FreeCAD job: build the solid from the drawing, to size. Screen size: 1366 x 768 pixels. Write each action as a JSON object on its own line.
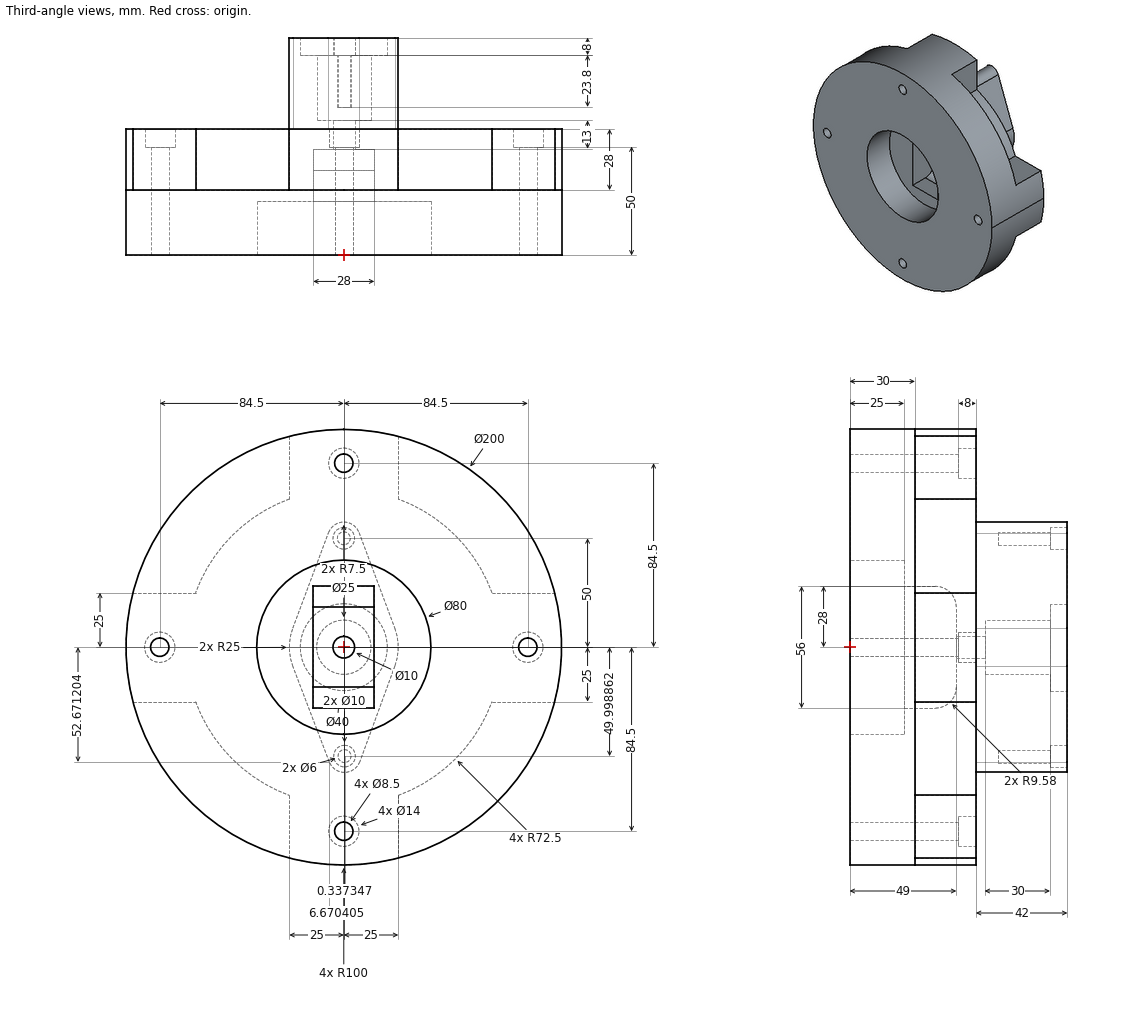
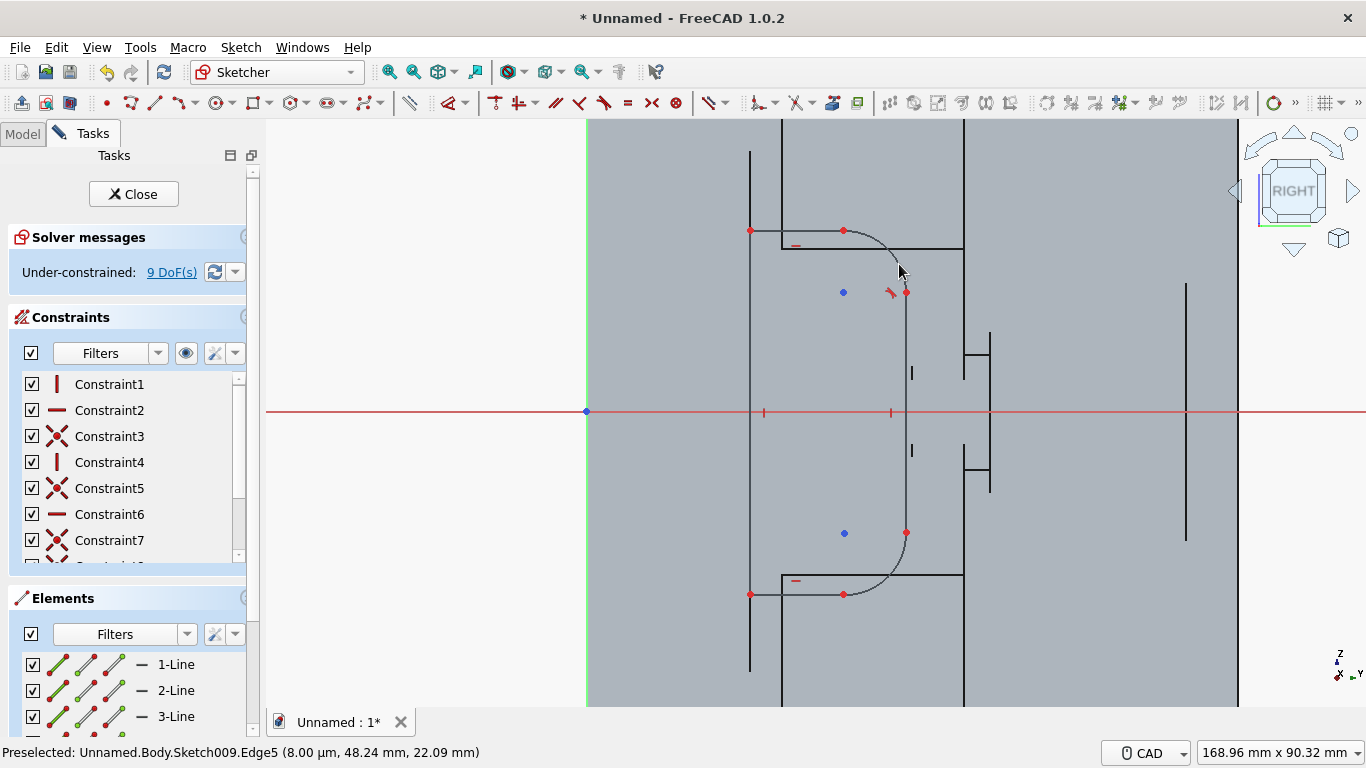
{"action": "left_click", "coordinate": [906, 461]}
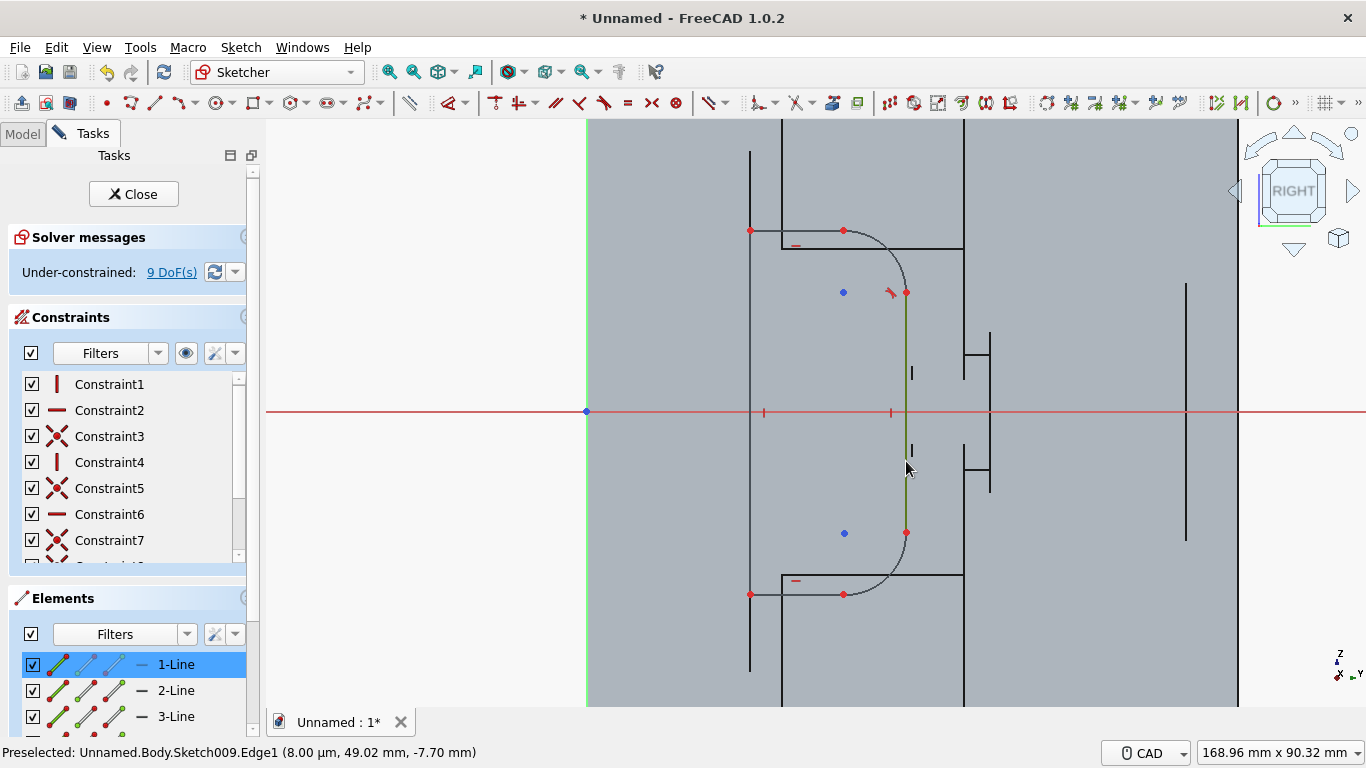
{"action": "left_click", "coordinate": [872, 589]}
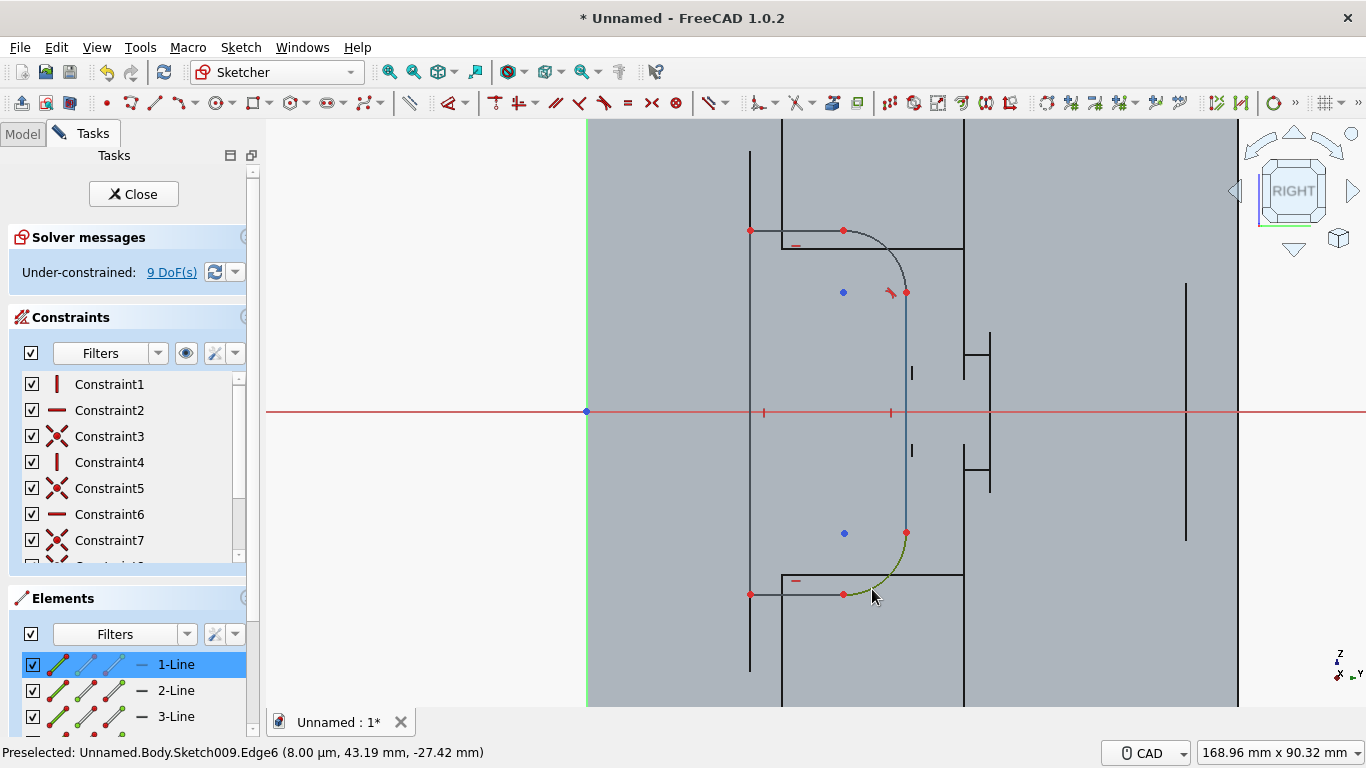
{"action": "left_click", "coordinate": [604, 104]}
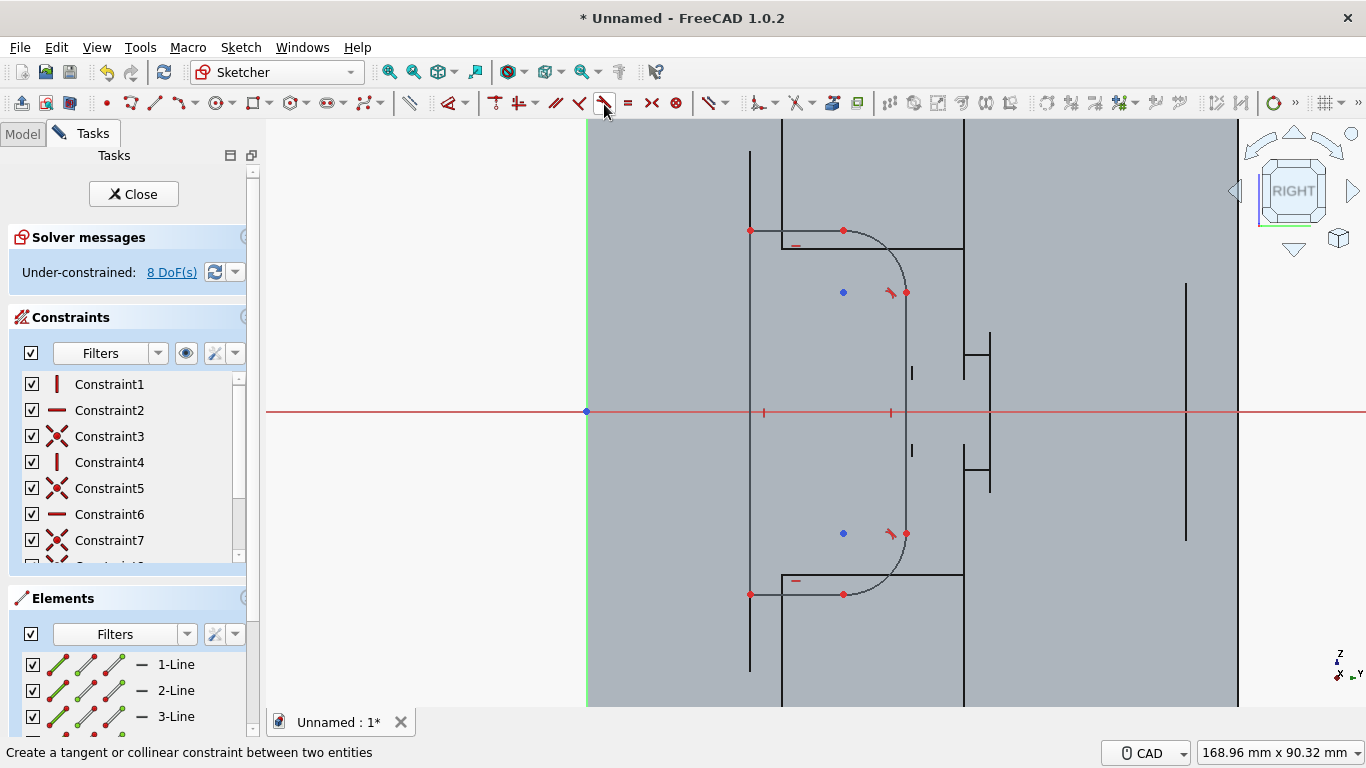
{"action": "left_click", "coordinate": [815, 231]}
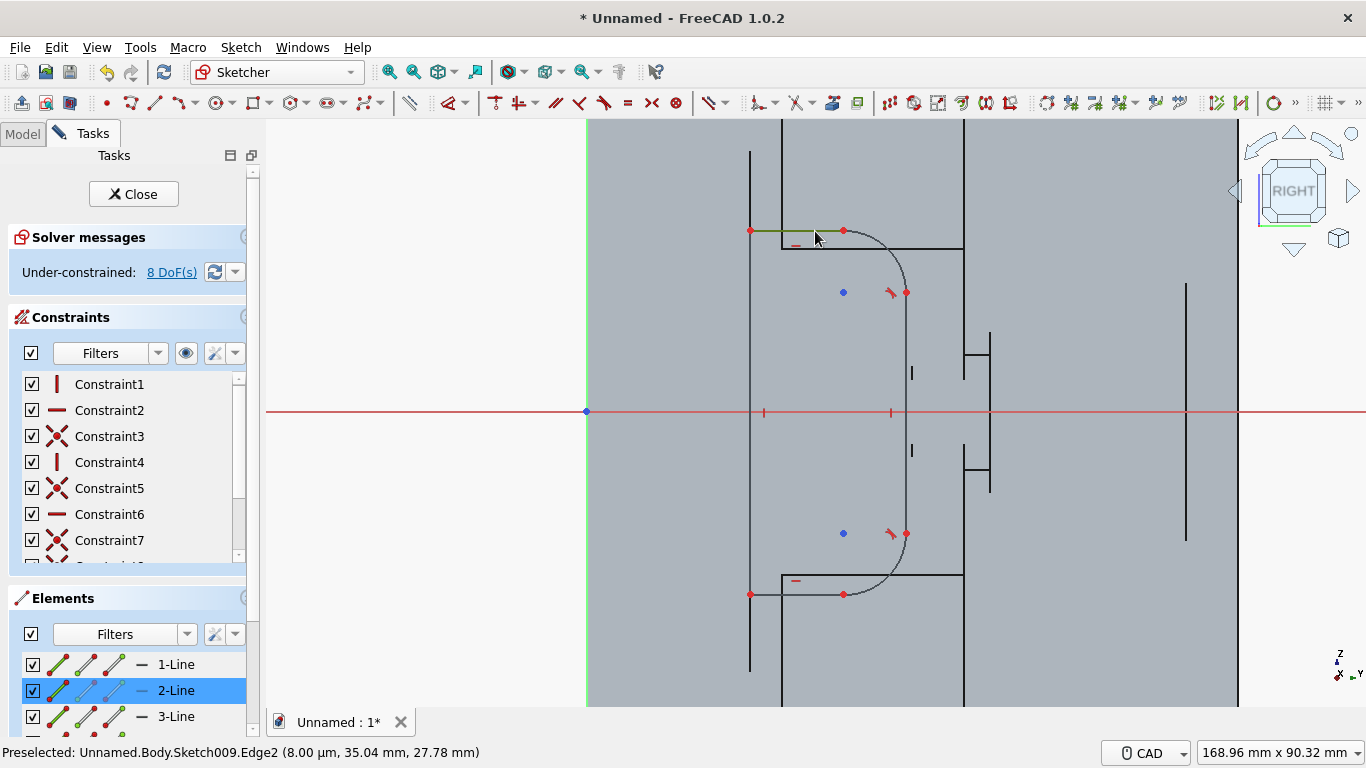
{"action": "left_click", "coordinate": [899, 265]}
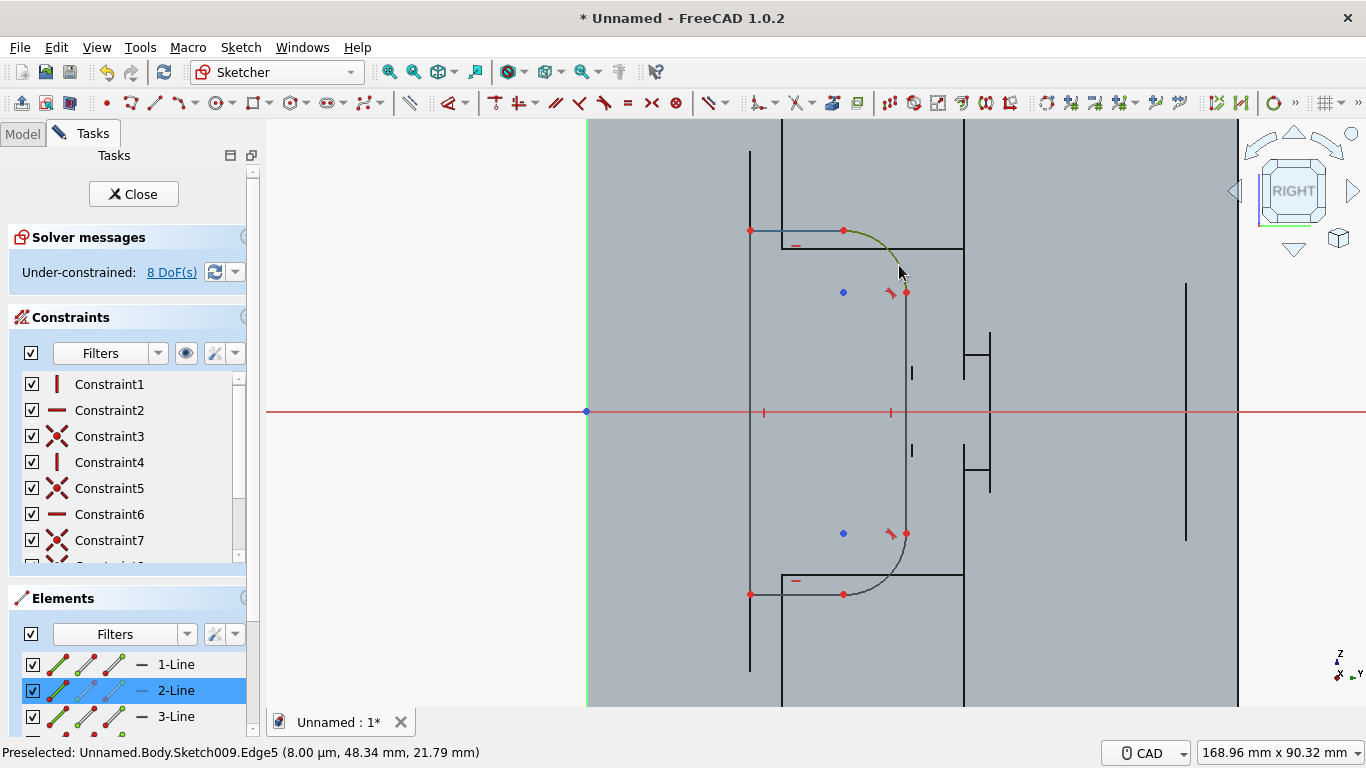
{"action": "key", "text": "t"}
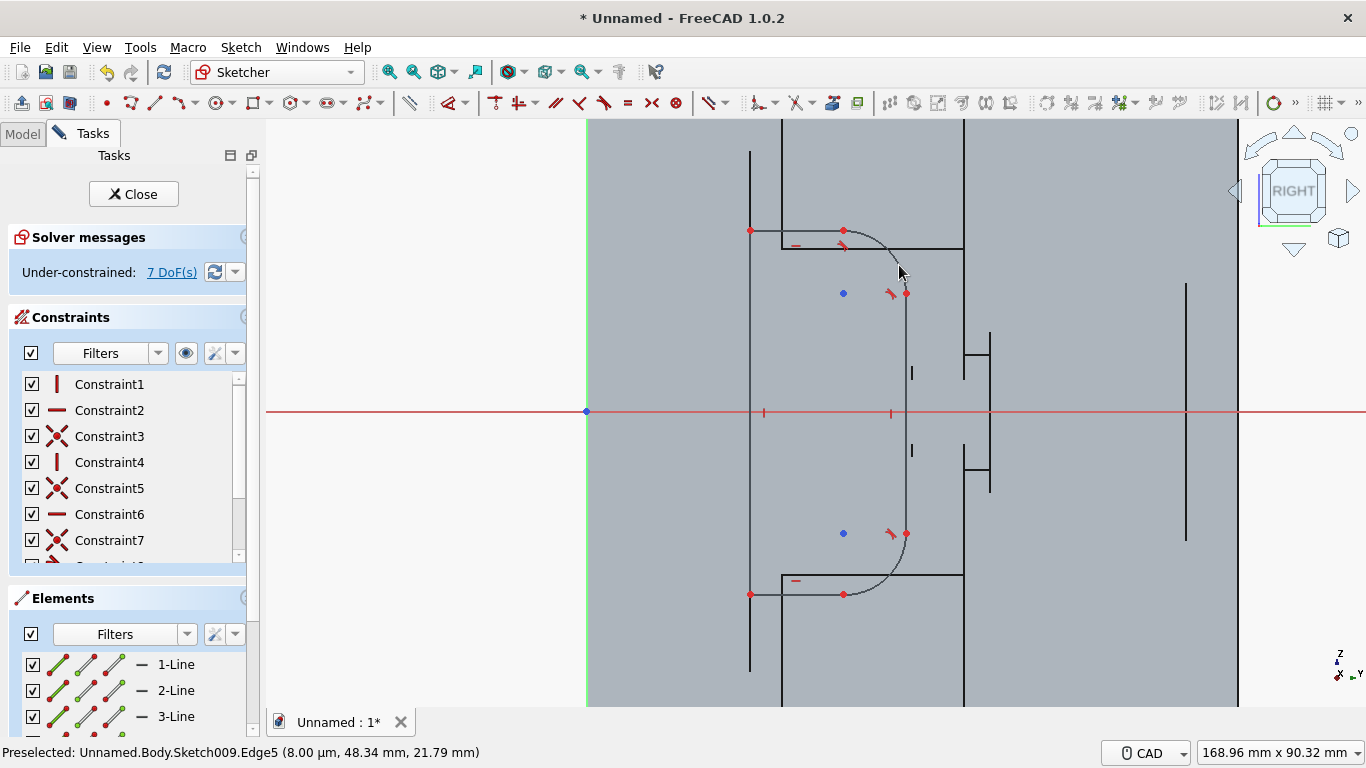
{"action": "left_click", "coordinate": [778, 595]}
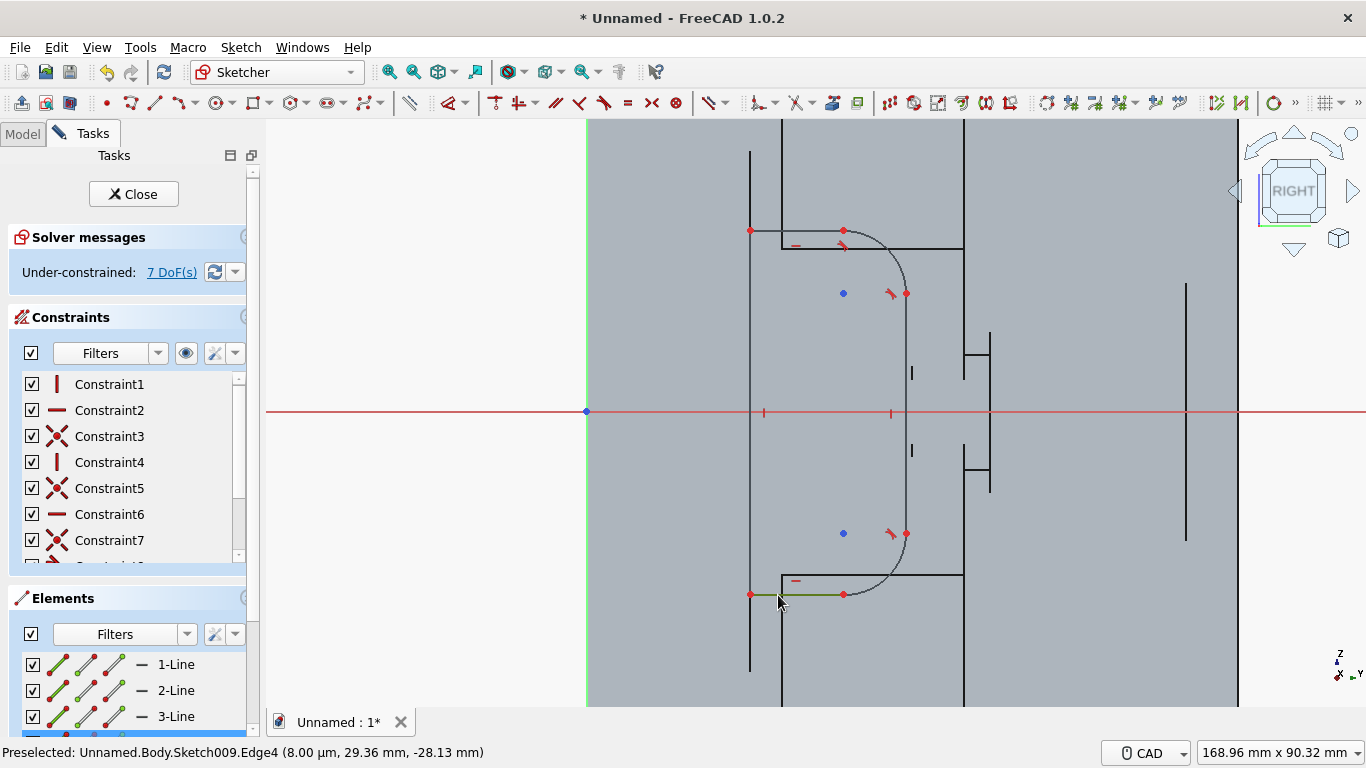
{"action": "left_click", "coordinate": [872, 589]}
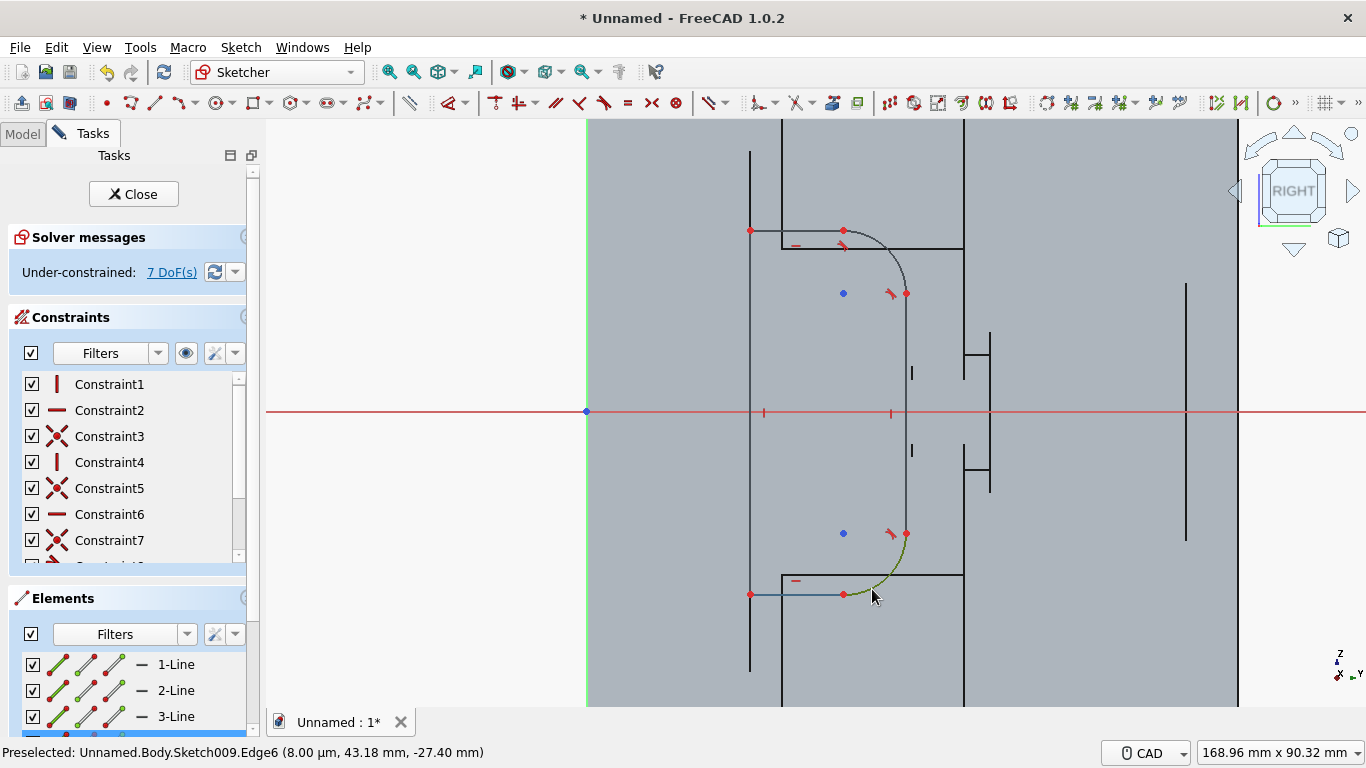
{"action": "key", "text": "t"}